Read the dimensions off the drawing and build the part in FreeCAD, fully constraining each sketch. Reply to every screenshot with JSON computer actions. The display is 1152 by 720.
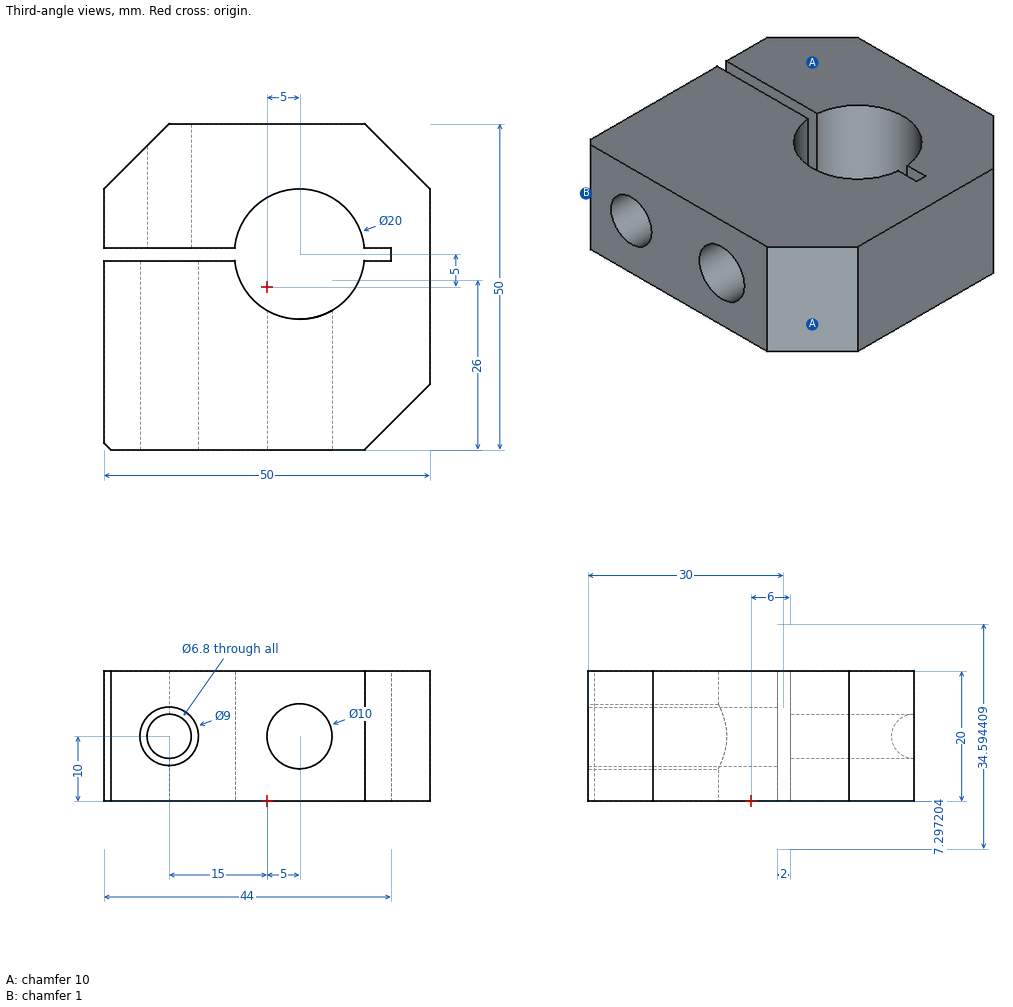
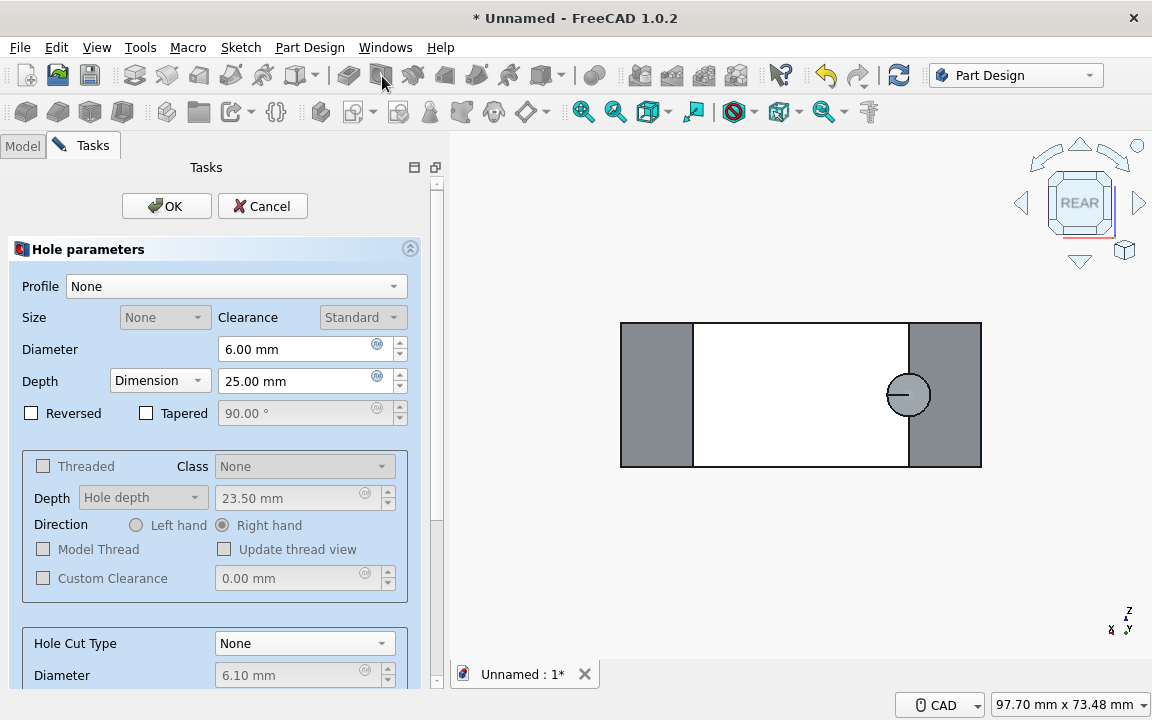
{"action": "triple_click", "coordinate": [305, 349]}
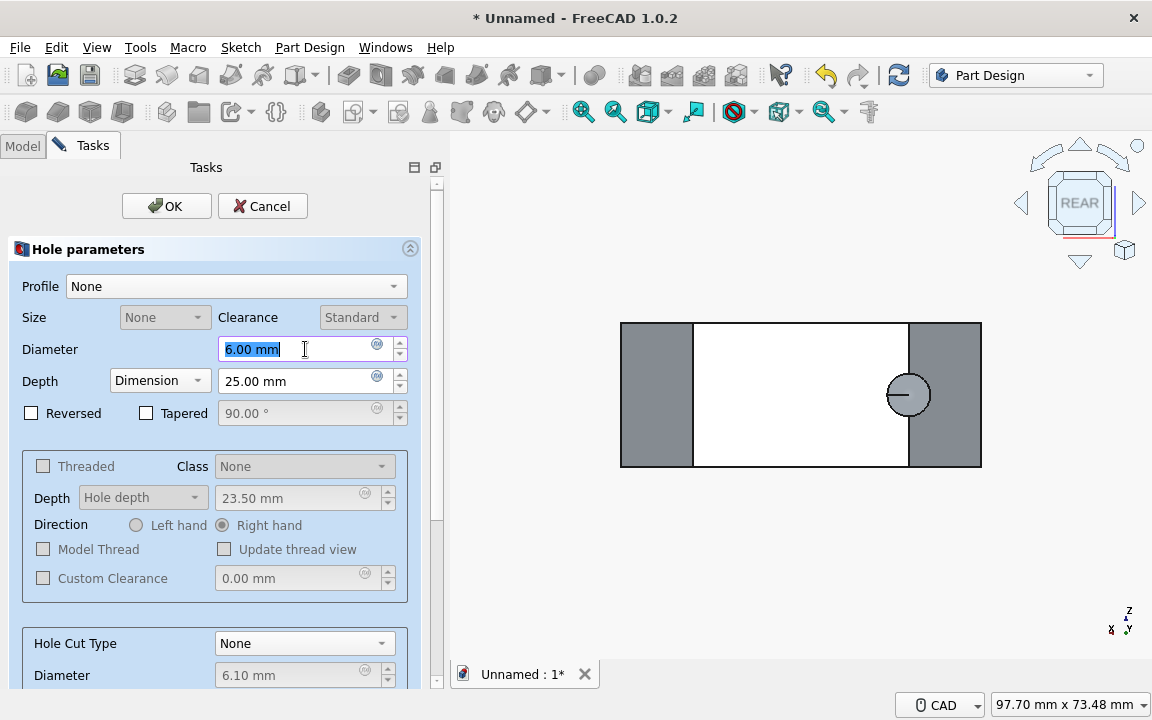
{"action": "type", "text": "6.8"}
{"action": "key", "text": "Tab"}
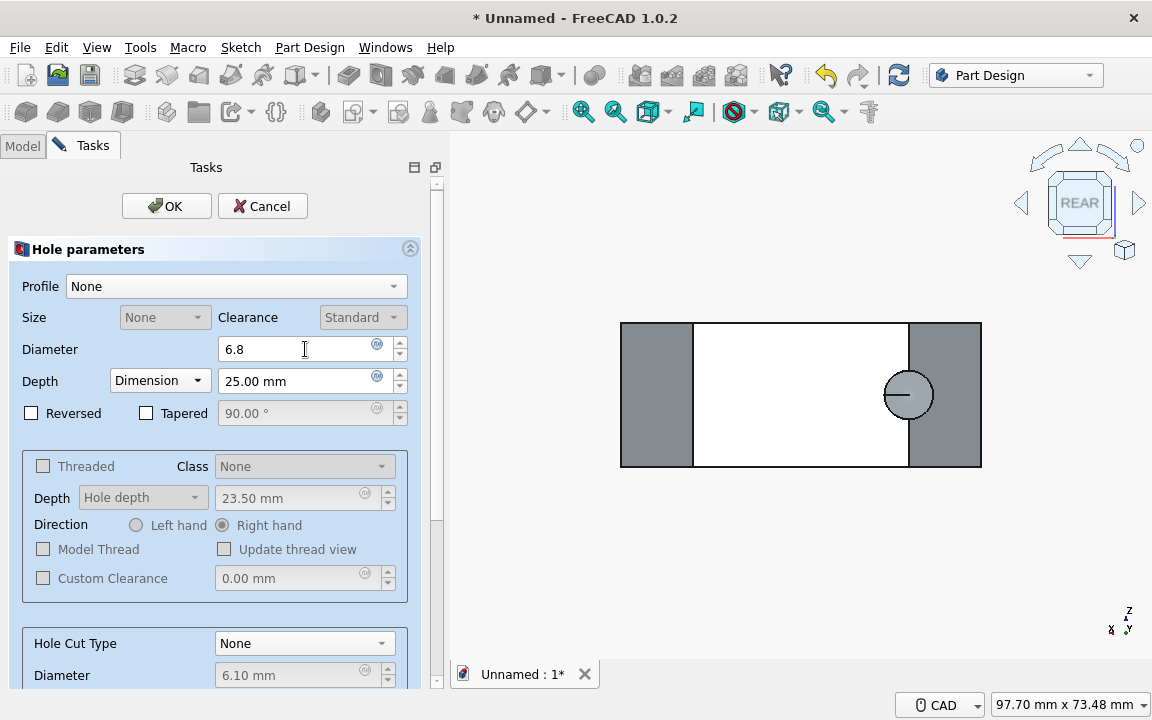
{"action": "left_click", "coordinate": [161, 380]}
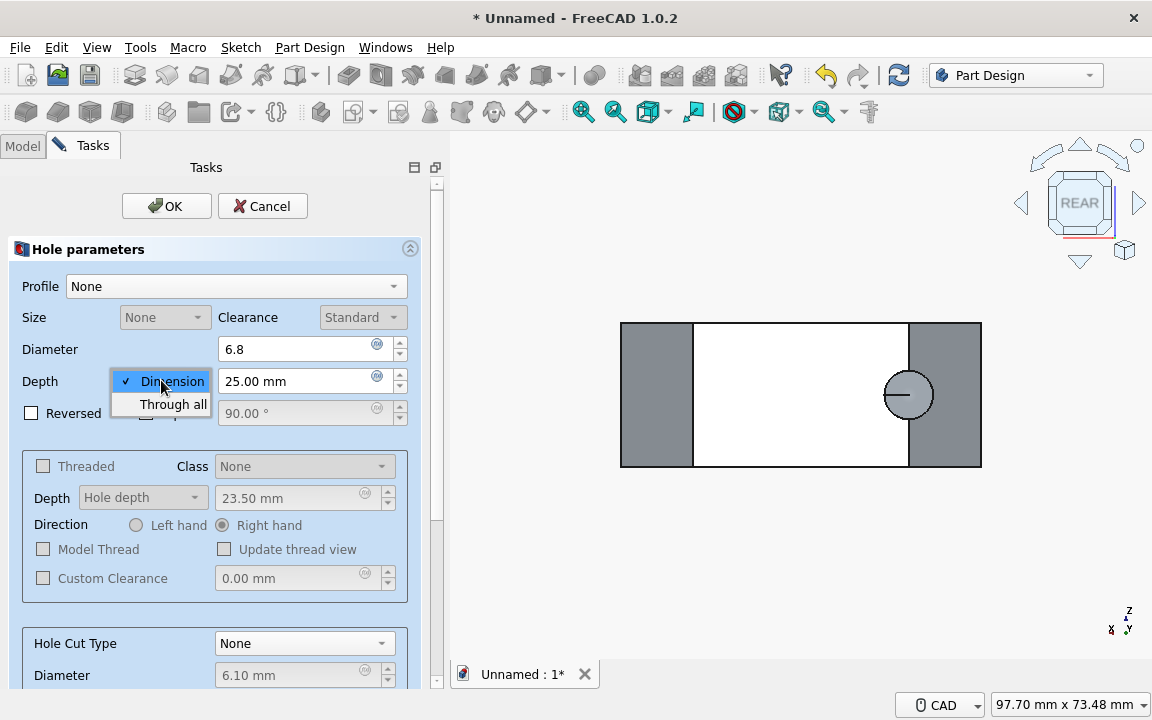
{"action": "left_click", "coordinate": [160, 404]}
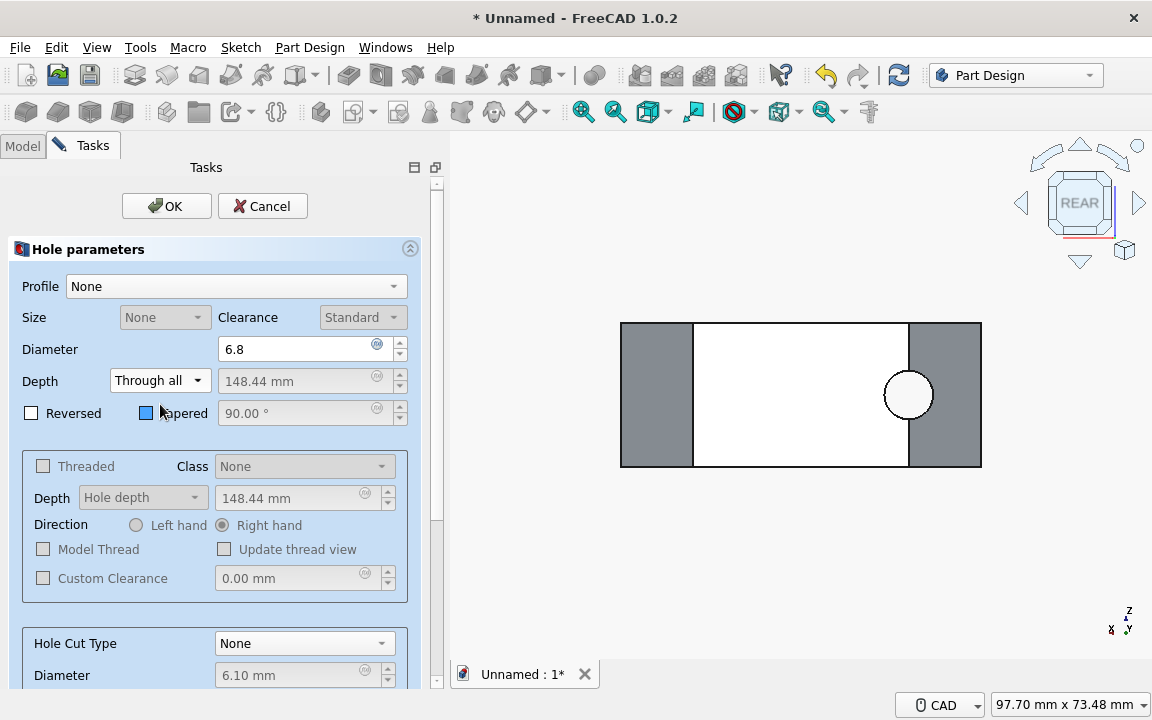
{"action": "left_click", "coordinate": [167, 206]}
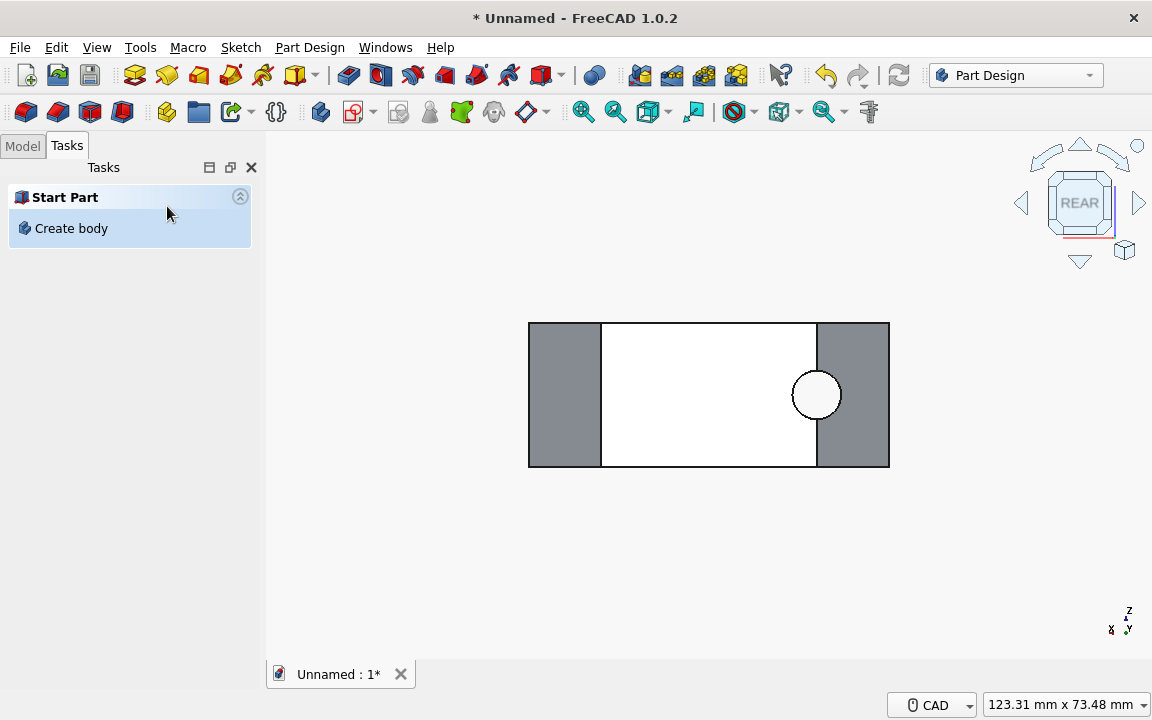
{"action": "left_click", "coordinate": [584, 112]}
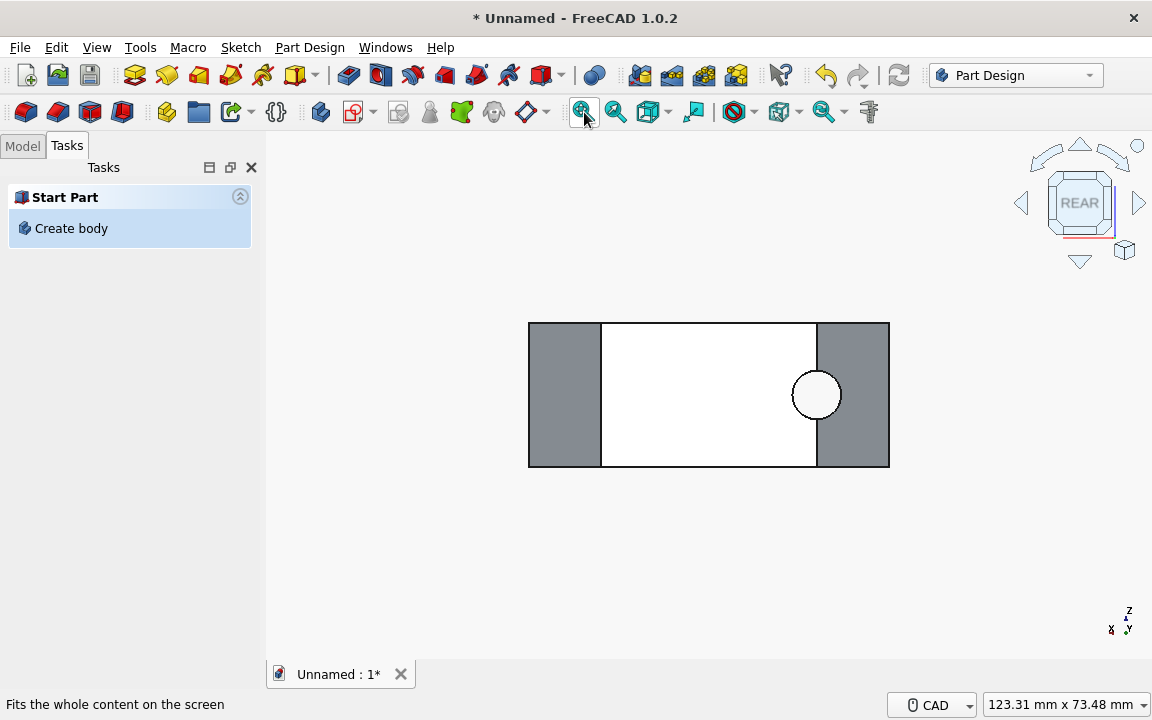
{"action": "key", "text": "0"}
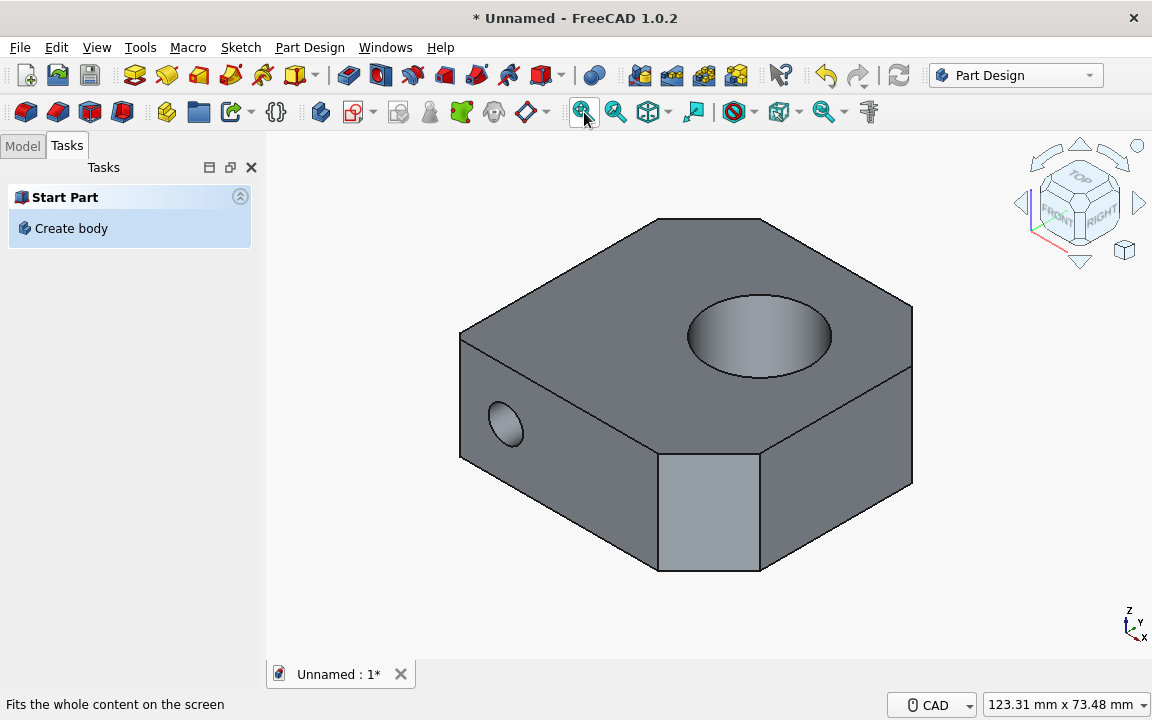
{"action": "left_click", "coordinate": [587, 470]}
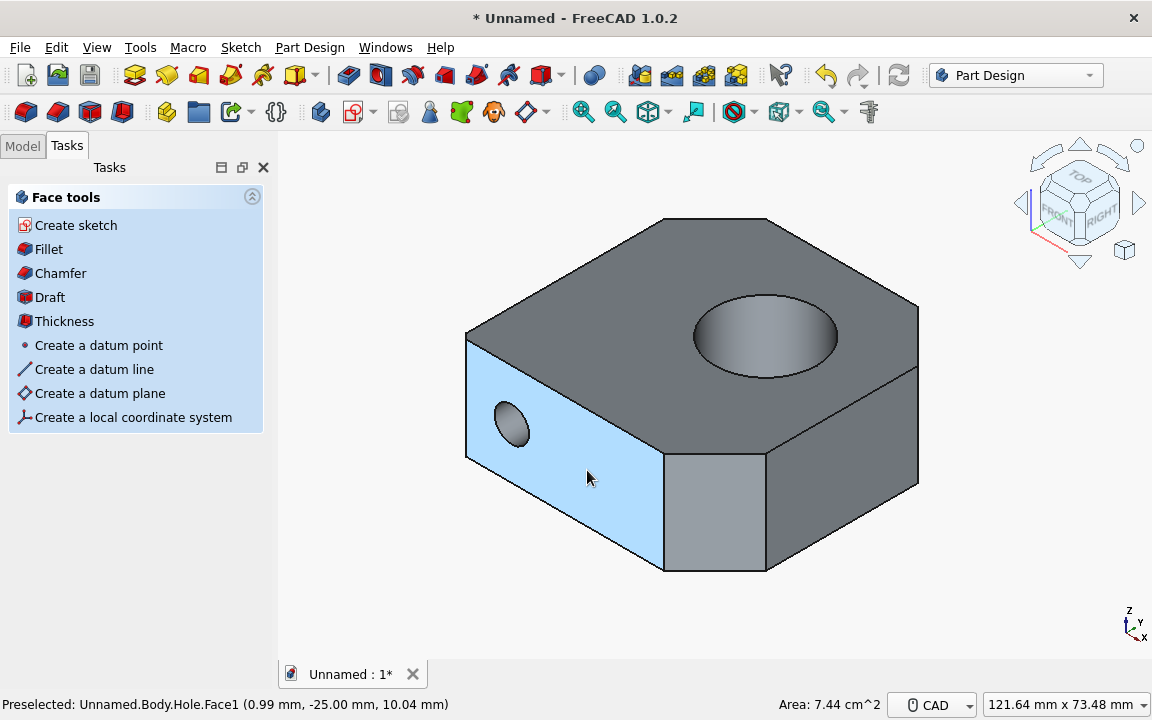
{"action": "left_click", "coordinate": [354, 112]}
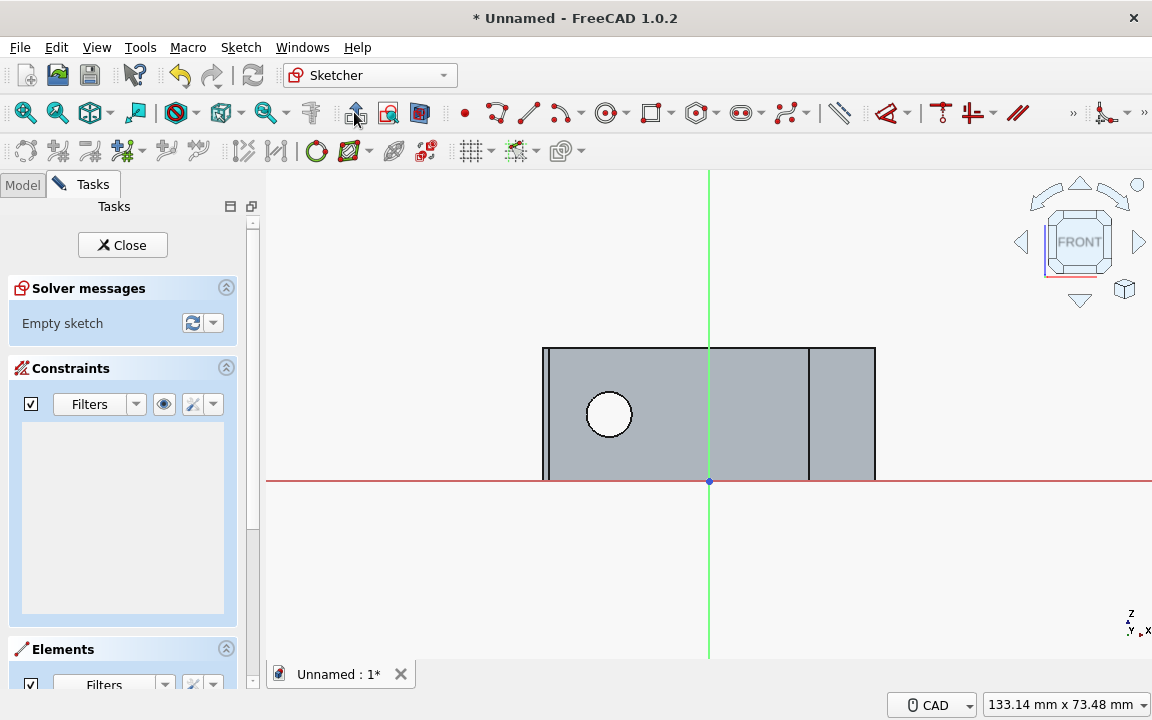
{"action": "scroll", "coordinate": [646, 441], "scroll_direction": "up", "scroll_amount": 6}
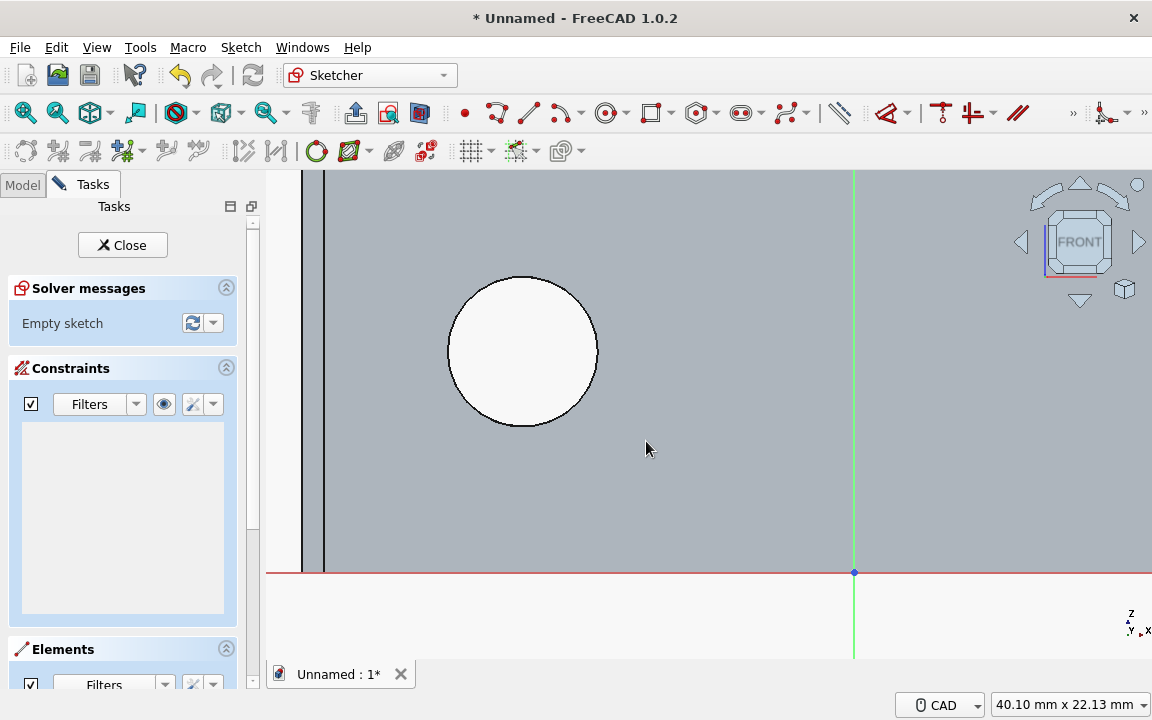
{"action": "left_click", "coordinate": [606, 114]}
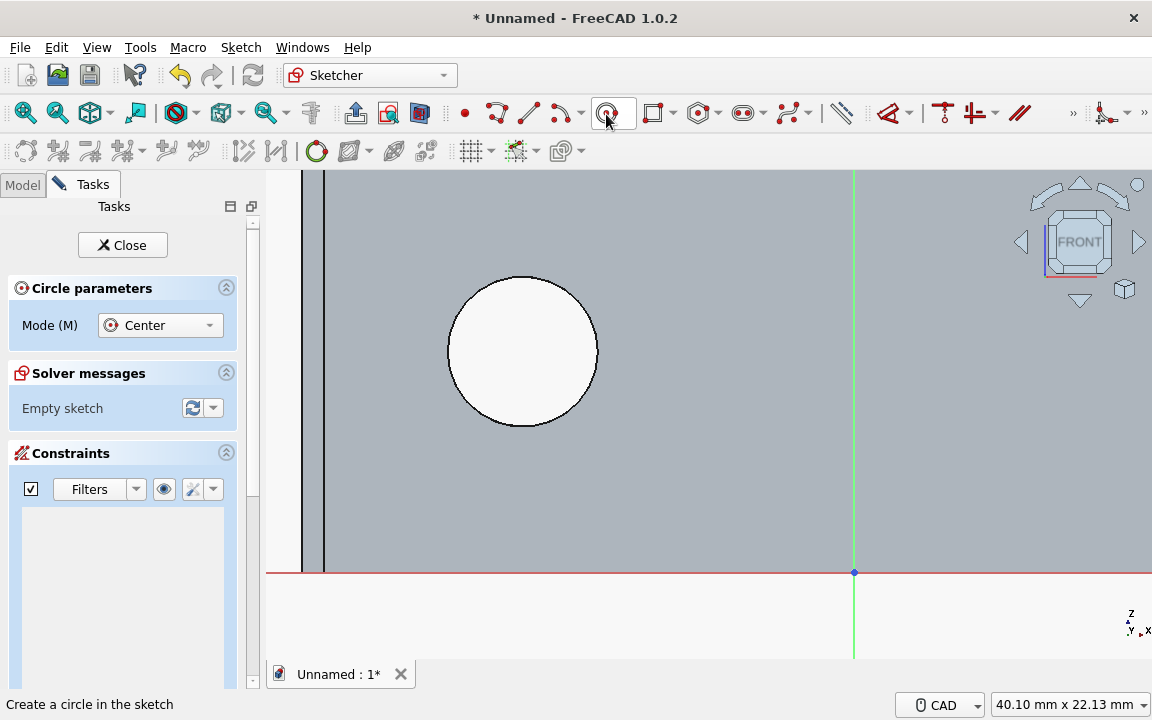
{"action": "left_click", "coordinate": [523, 352]}
{"action": "mouse_move", "coordinate": [593, 281]}